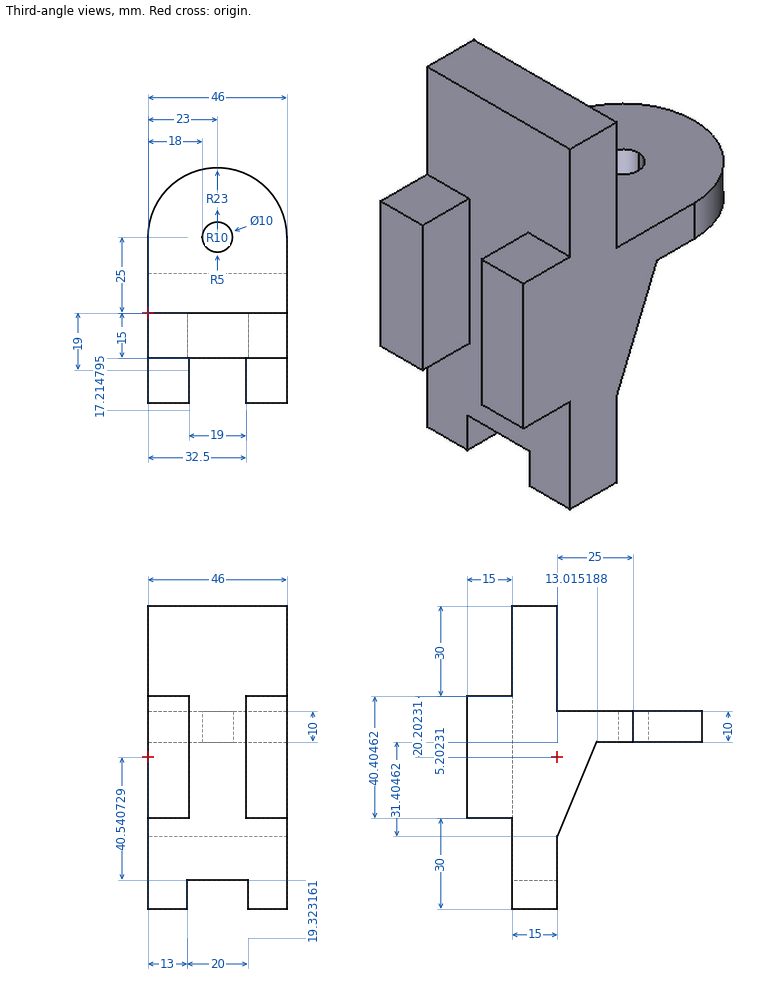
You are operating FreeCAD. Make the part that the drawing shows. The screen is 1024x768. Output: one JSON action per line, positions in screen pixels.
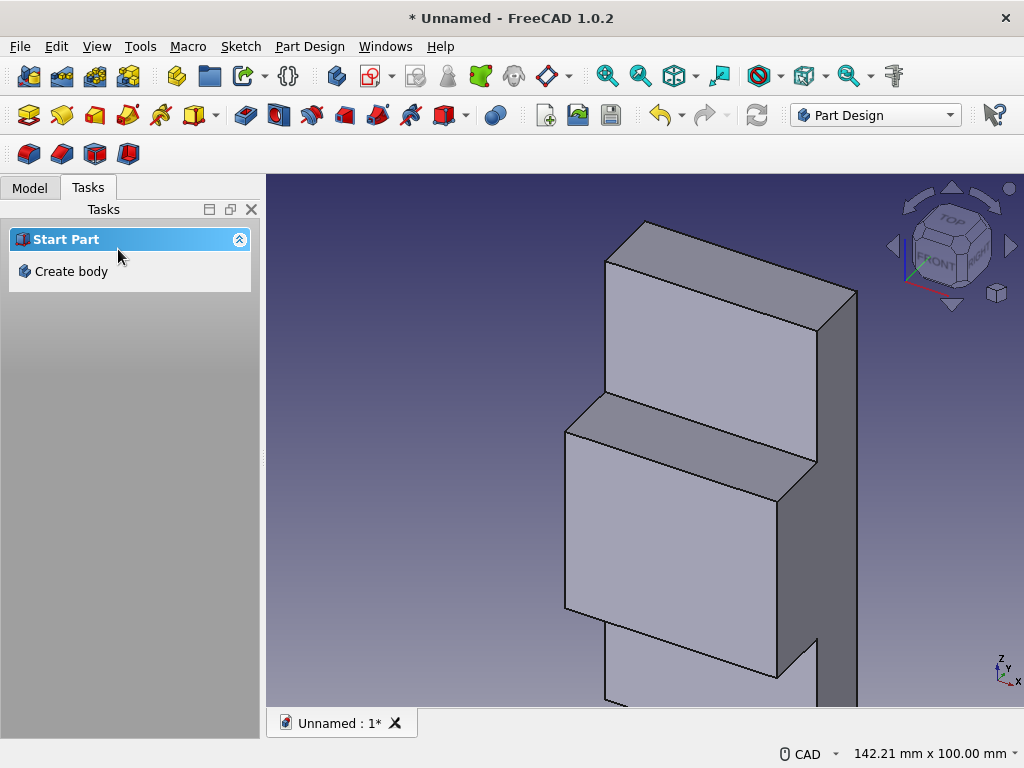
{"action": "key", "text": "v f"}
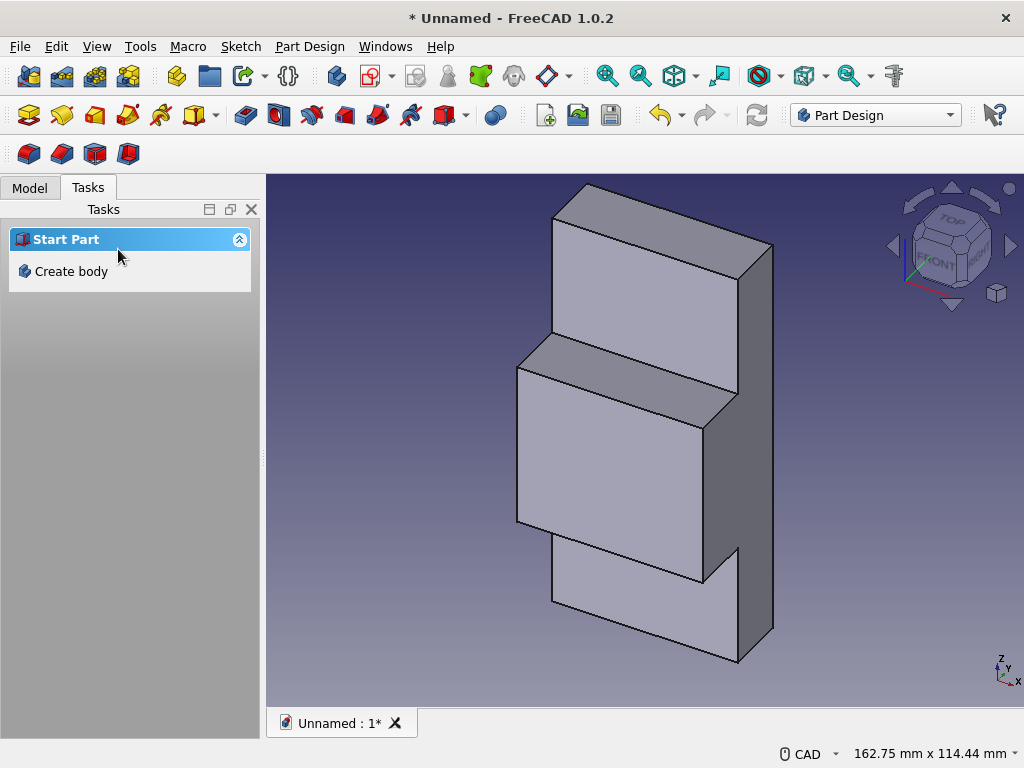
{"action": "left_click", "coordinate": [30, 188]}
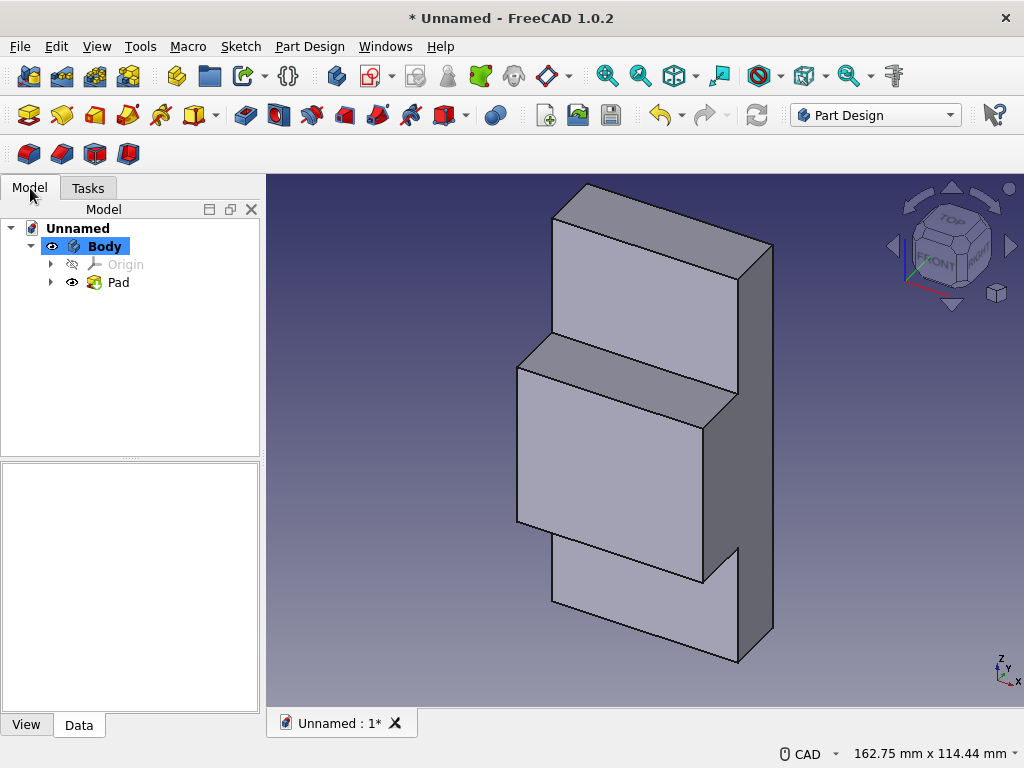
{"action": "left_click", "coordinate": [51, 264]}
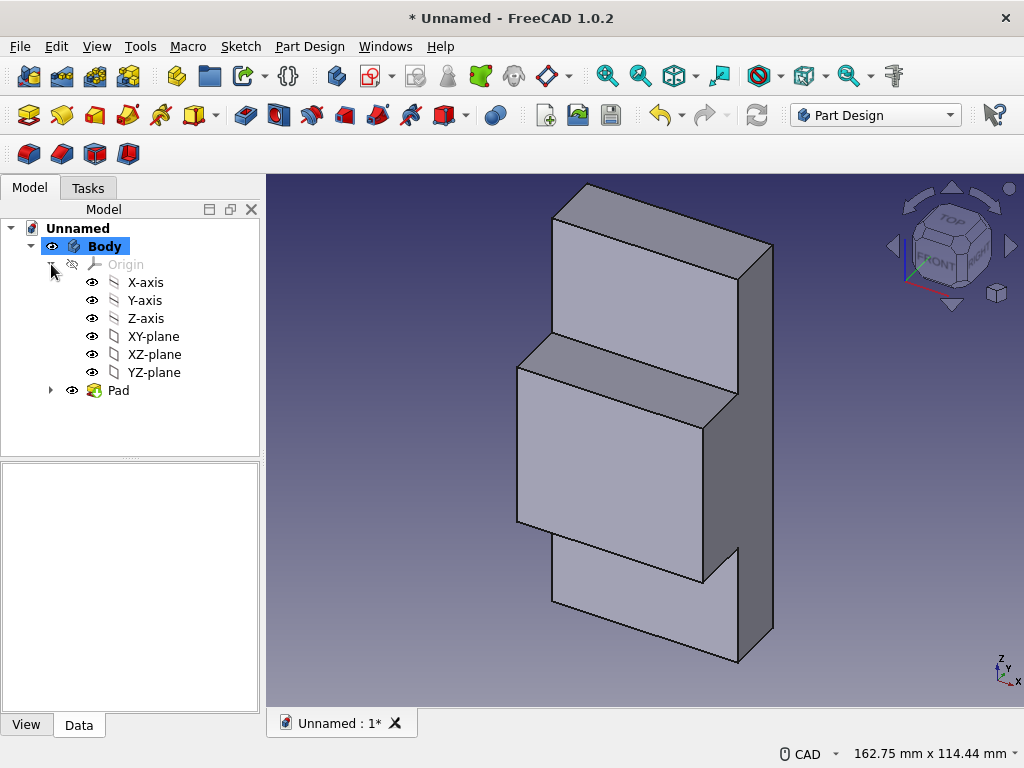
{"action": "left_click", "coordinate": [137, 372]}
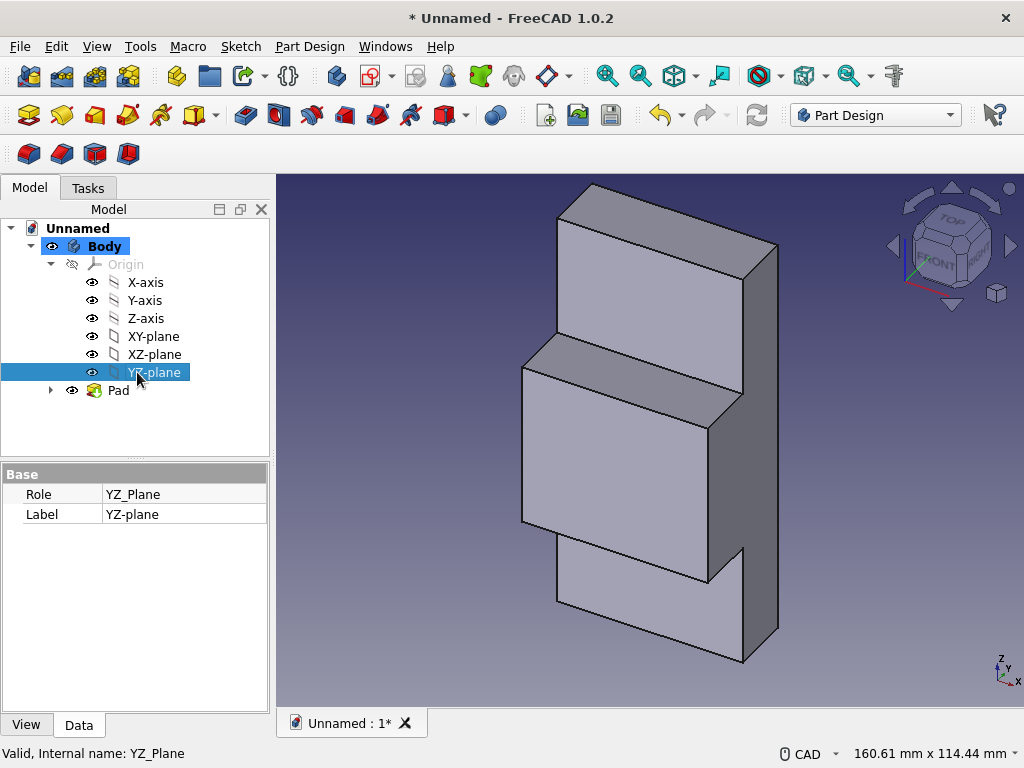
{"action": "left_click", "coordinate": [546, 76]}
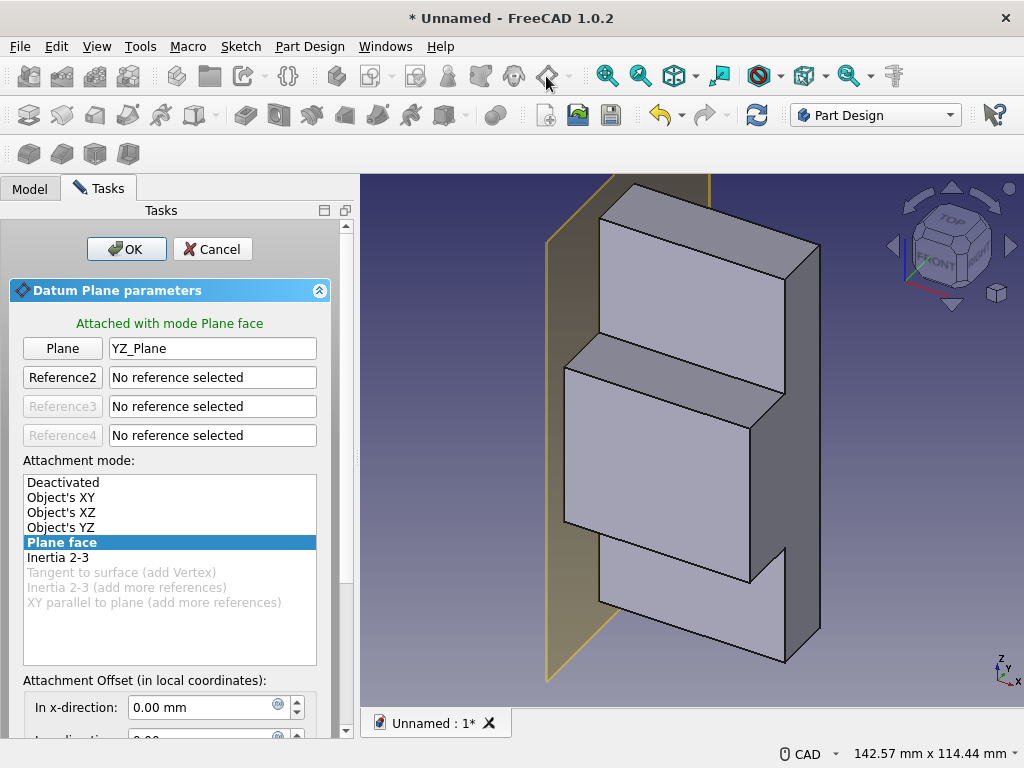
{"action": "scroll", "coordinate": [346, 479], "scroll_direction": "down", "scroll_amount": 2}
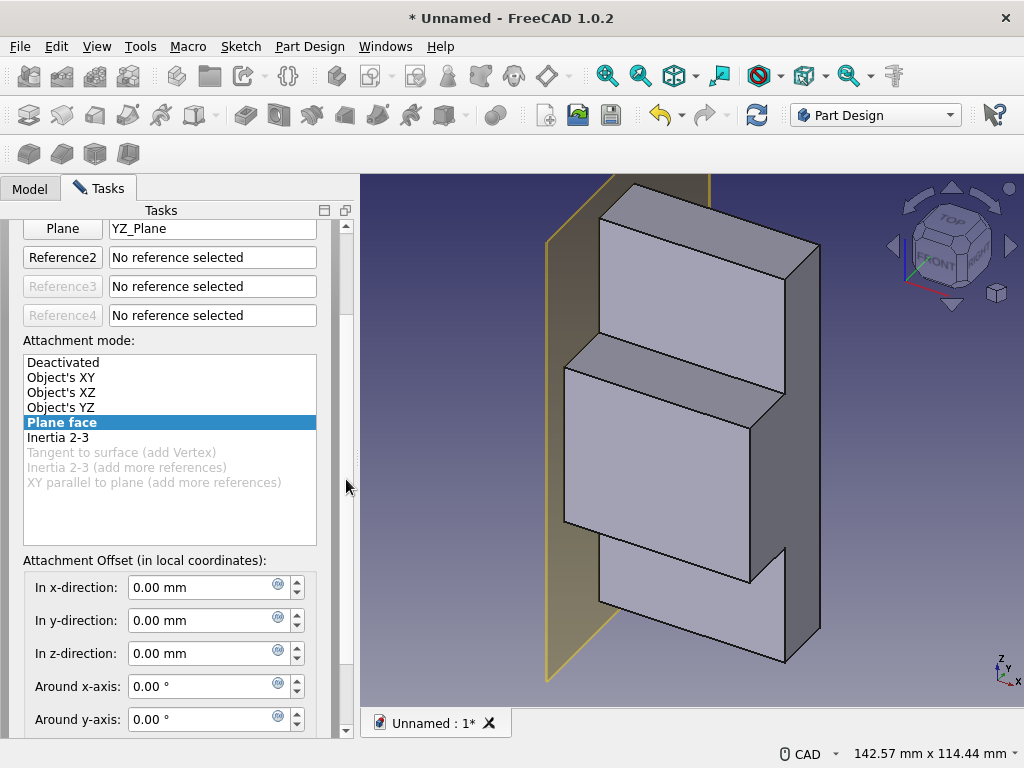
{"action": "triple_click", "coordinate": [210, 654]}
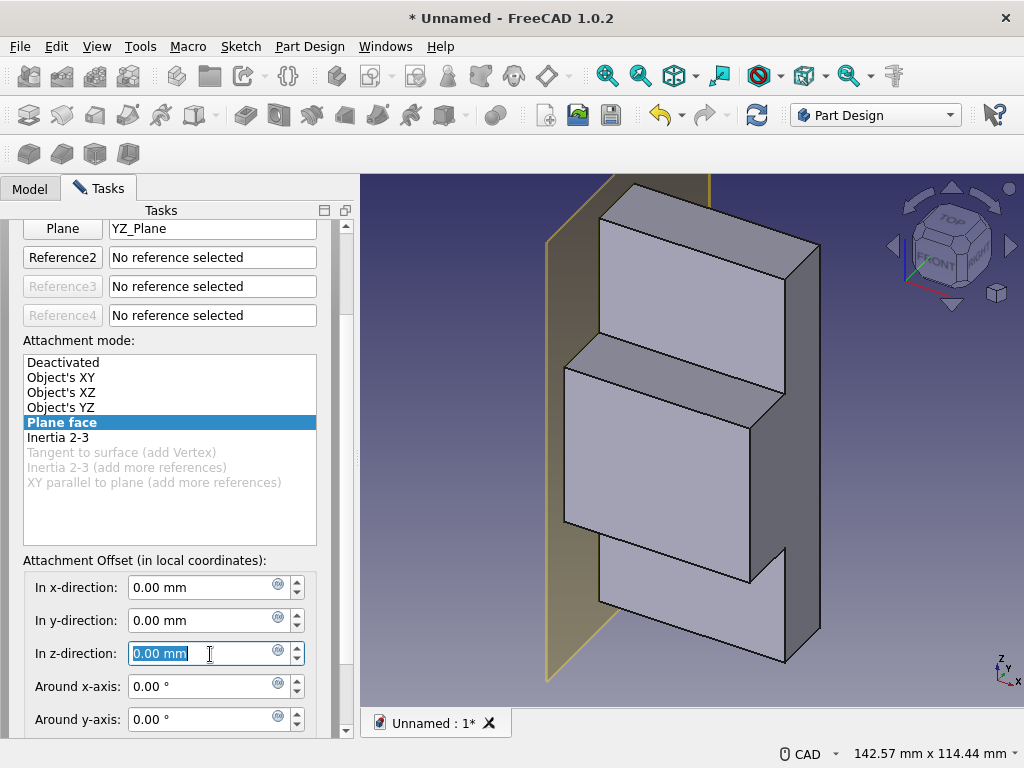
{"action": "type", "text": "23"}
{"action": "key", "text": "Tab"}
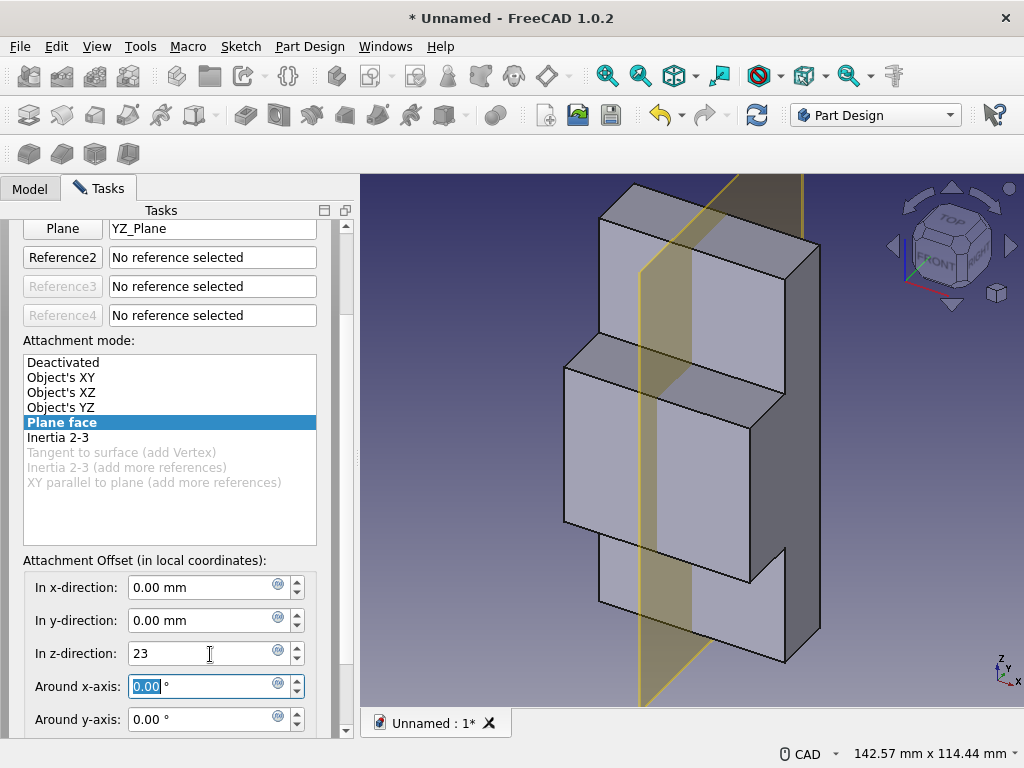
{"action": "scroll", "coordinate": [346, 479], "scroll_direction": "up", "scroll_amount": 3}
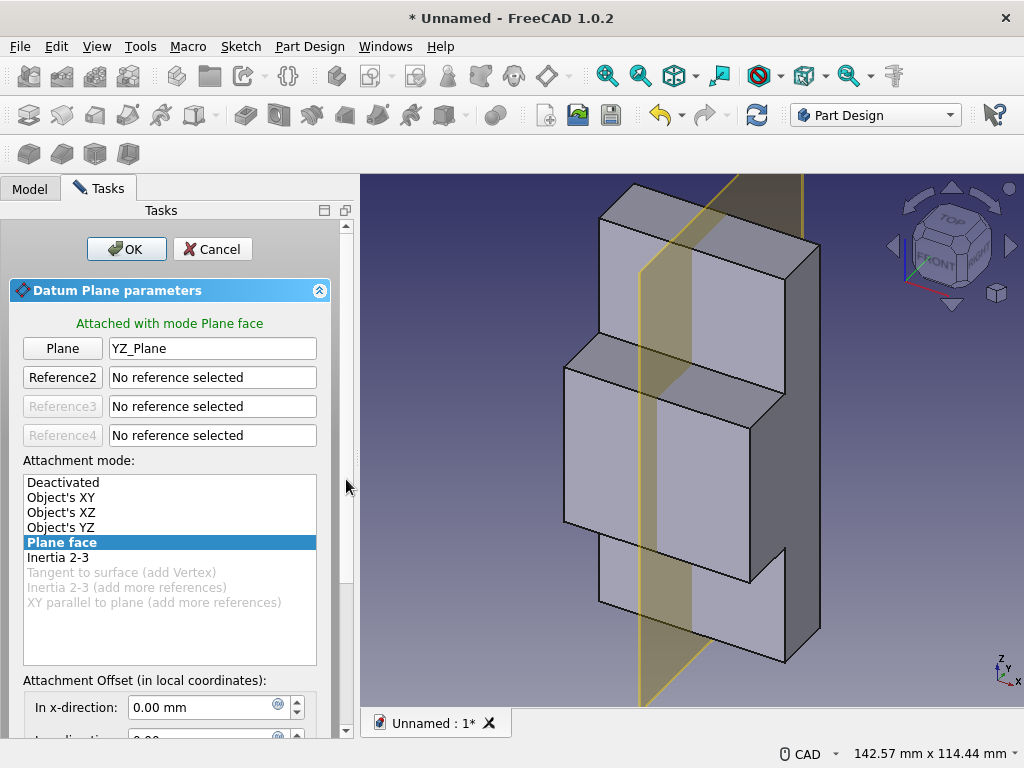
{"action": "left_click", "coordinate": [127, 249]}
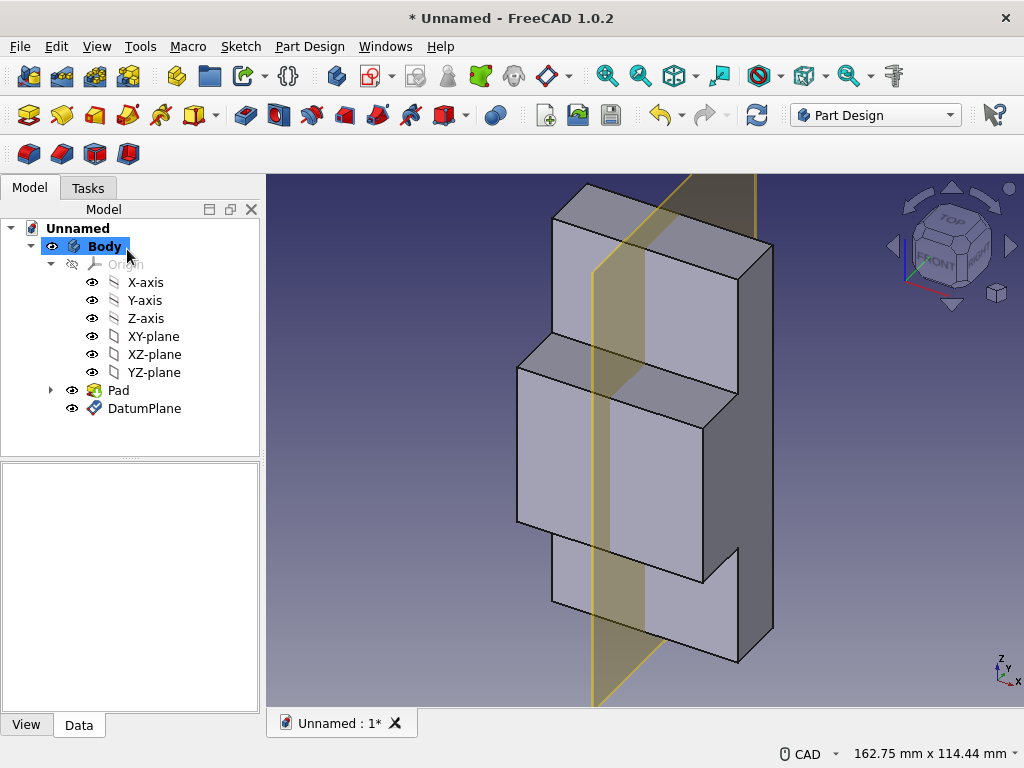
{"action": "left_click", "coordinate": [117, 408]}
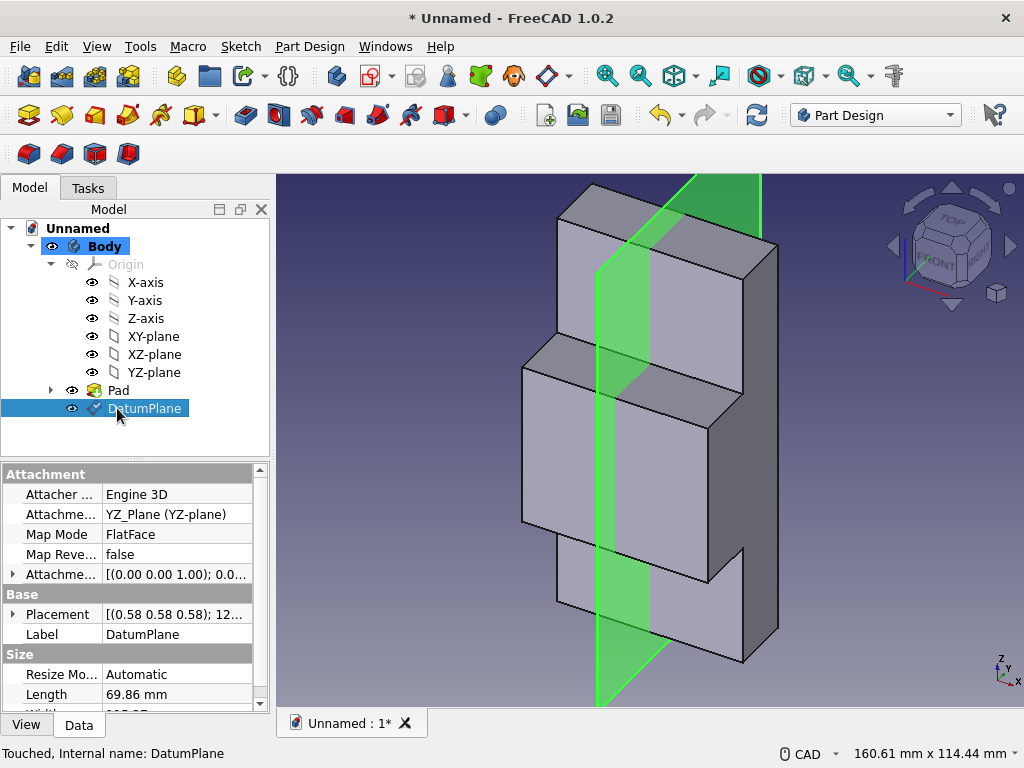
{"action": "left_click", "coordinate": [370, 76]}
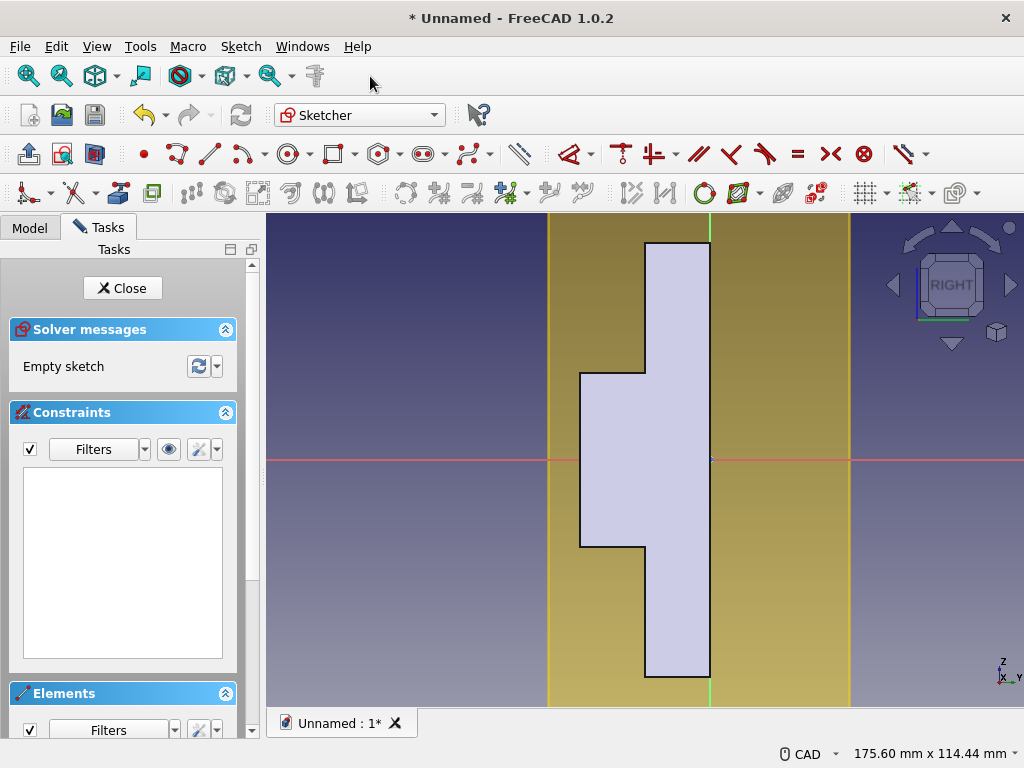
{"action": "left_click", "coordinate": [95, 154]}